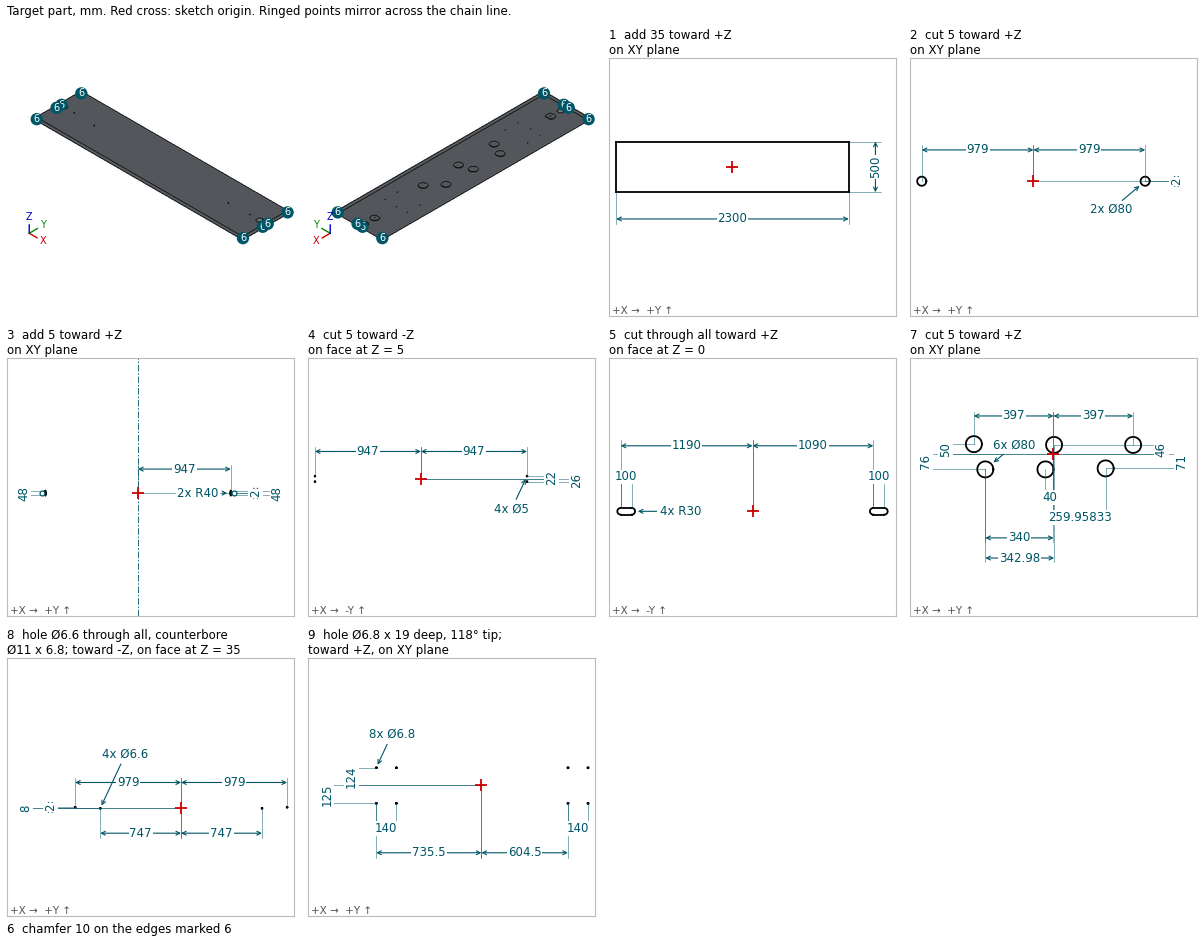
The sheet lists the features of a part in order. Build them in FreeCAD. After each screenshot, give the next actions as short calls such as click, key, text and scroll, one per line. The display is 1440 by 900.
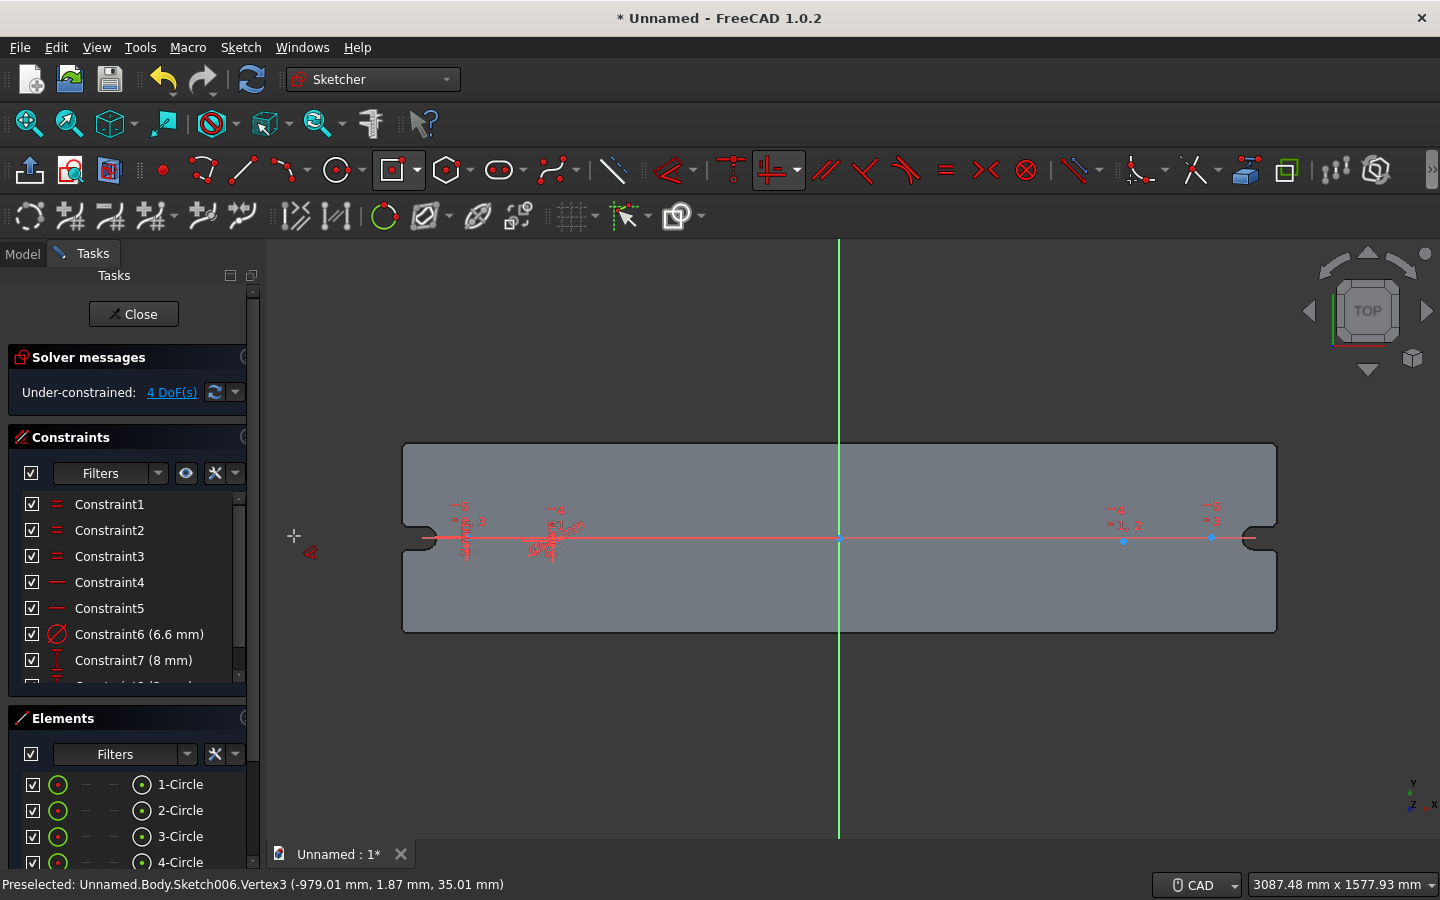
click(555, 541)
click(697, 575)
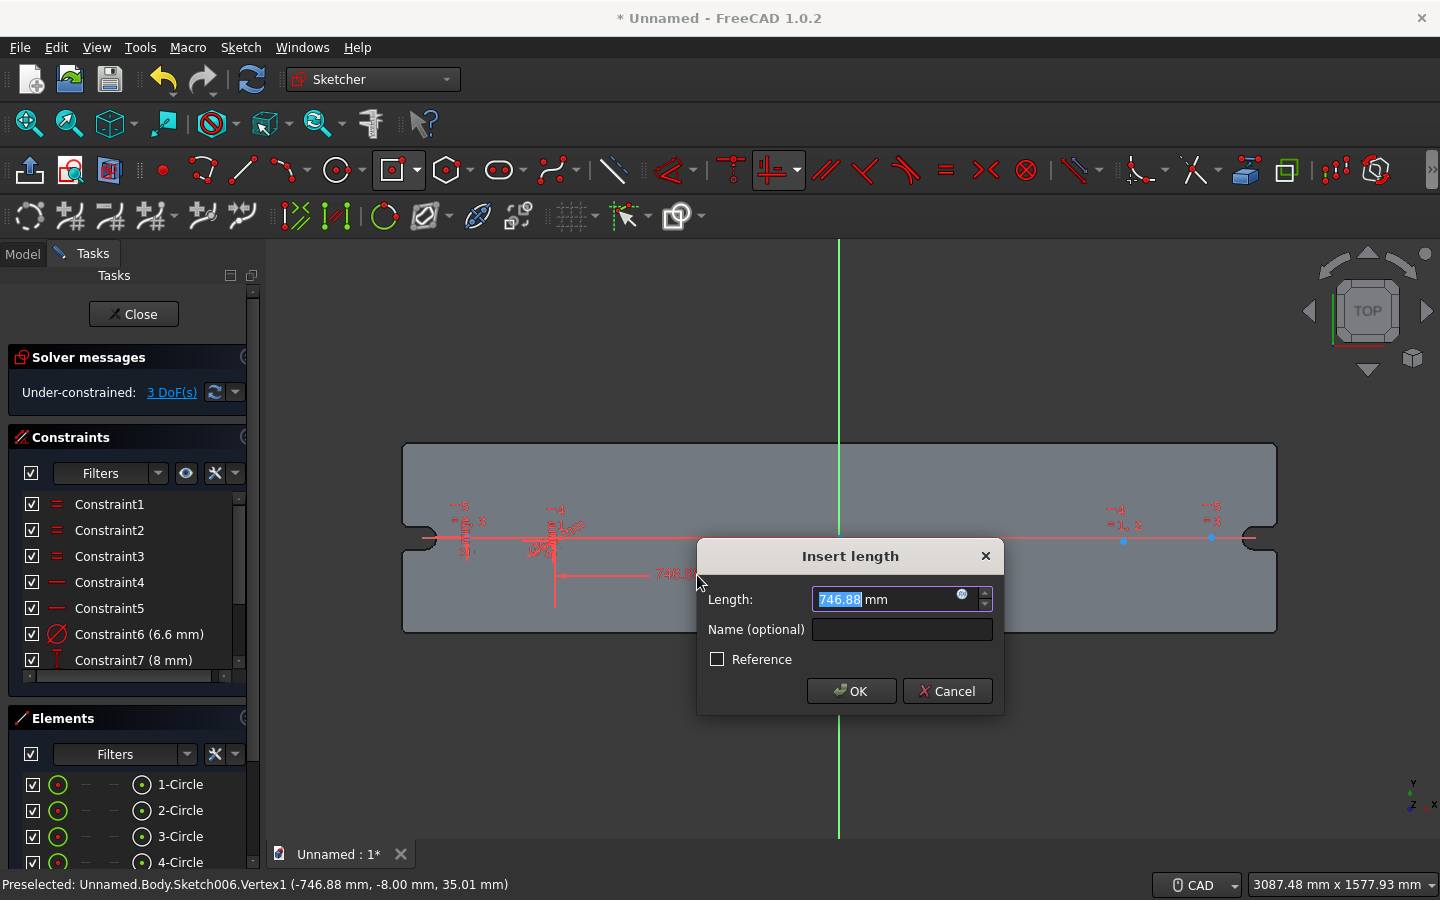
text(747)
key(Return)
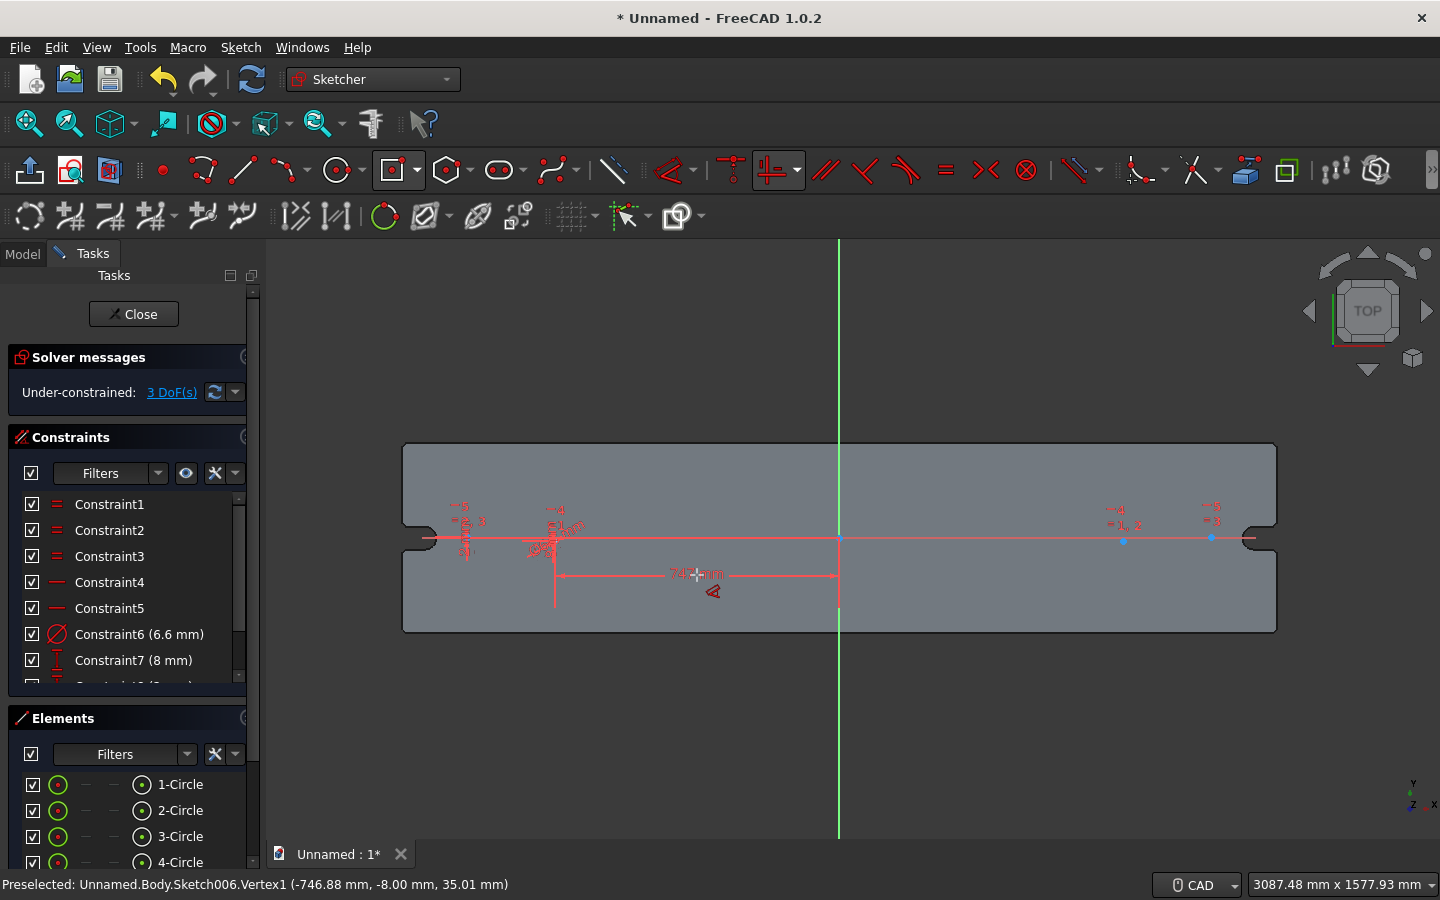
click(1123, 541)
click(981, 575)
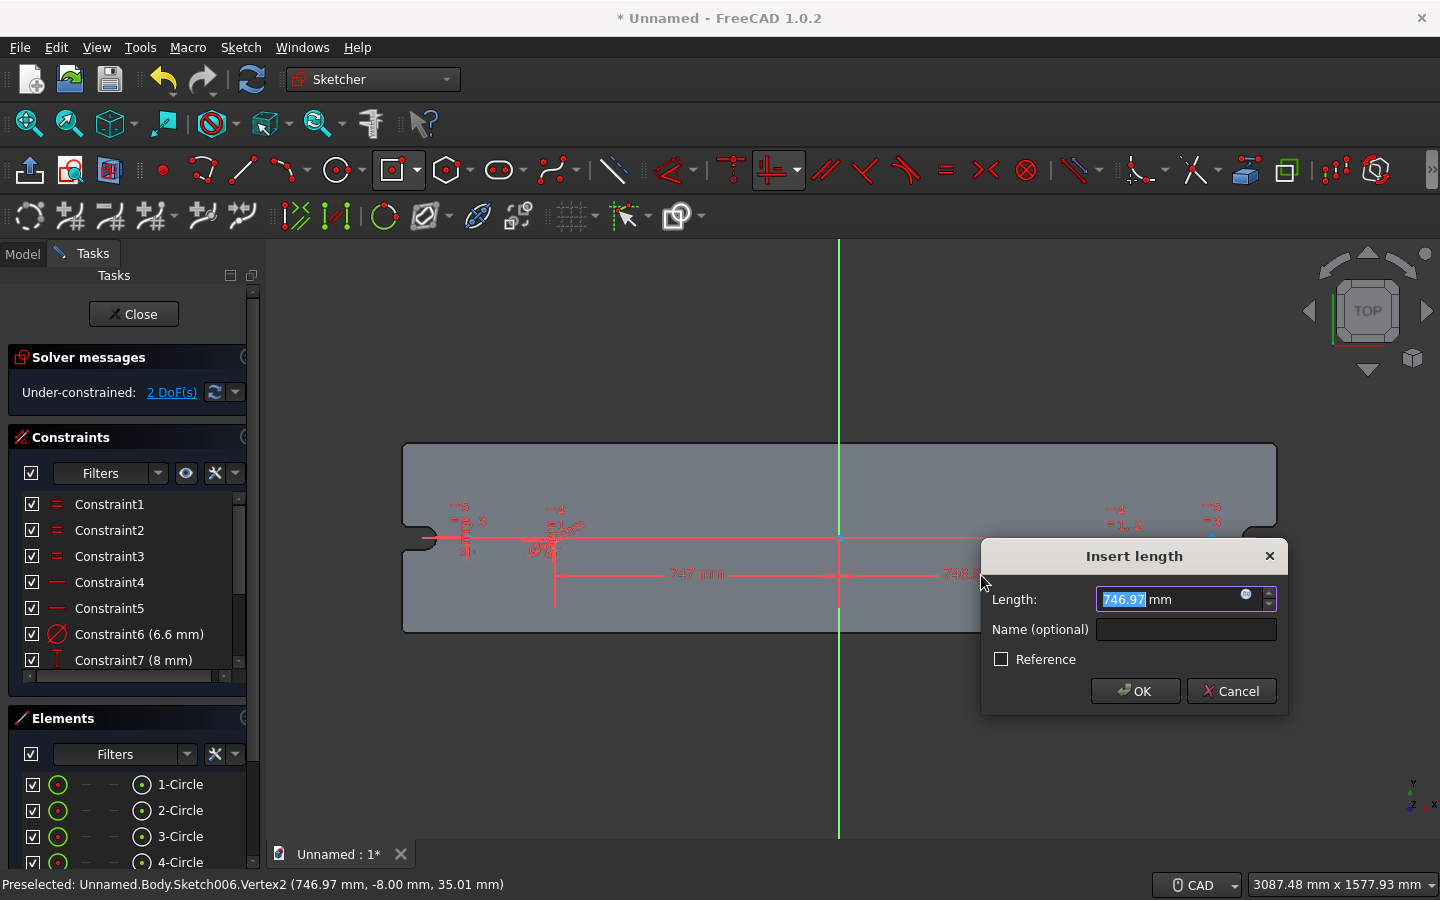
text(747)
key(Return)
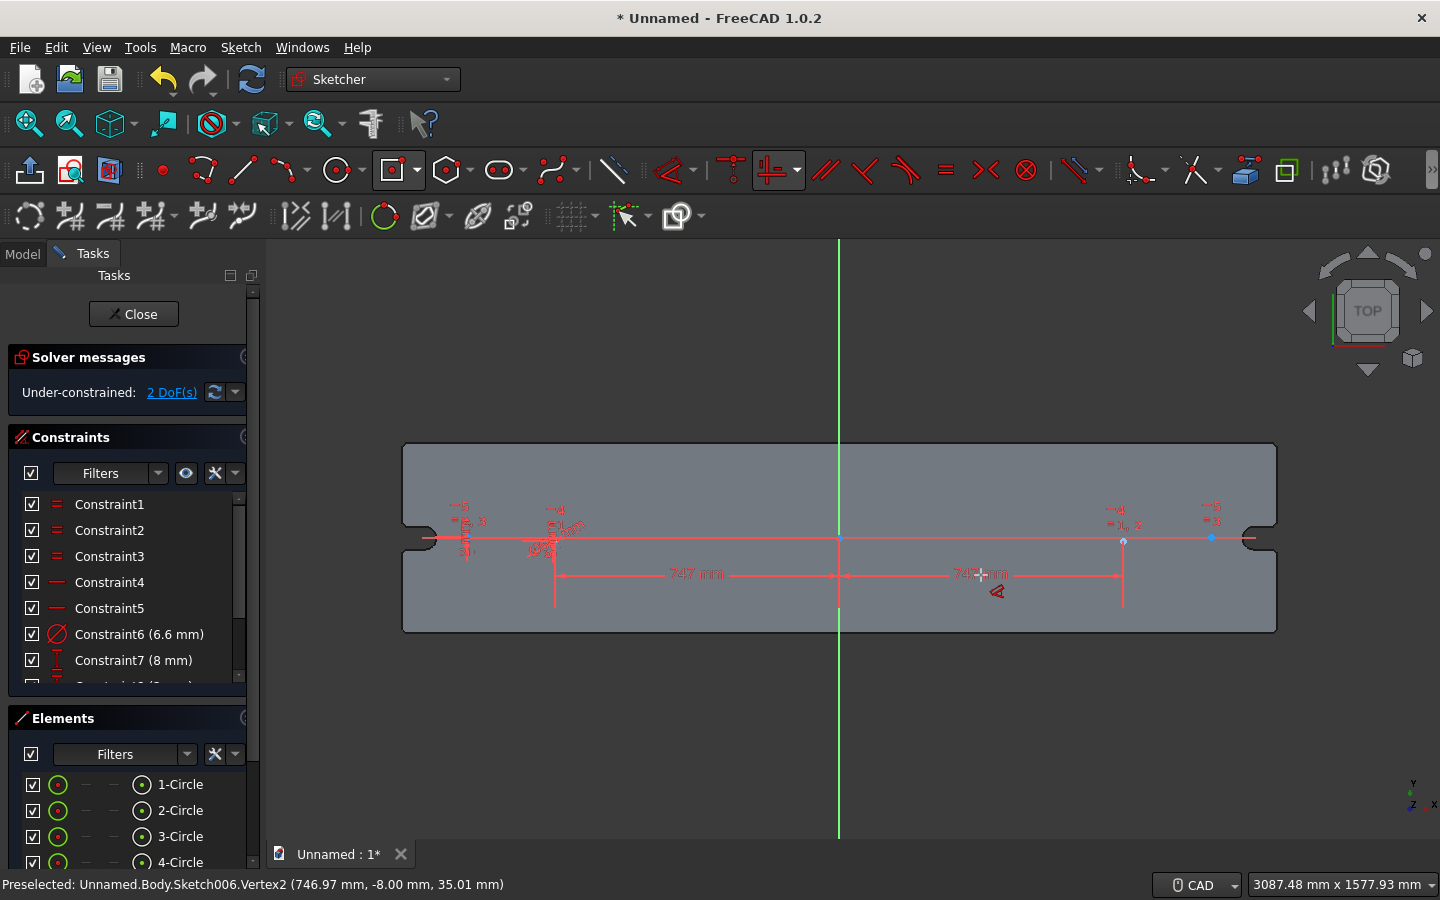
click(467, 537)
click(653, 503)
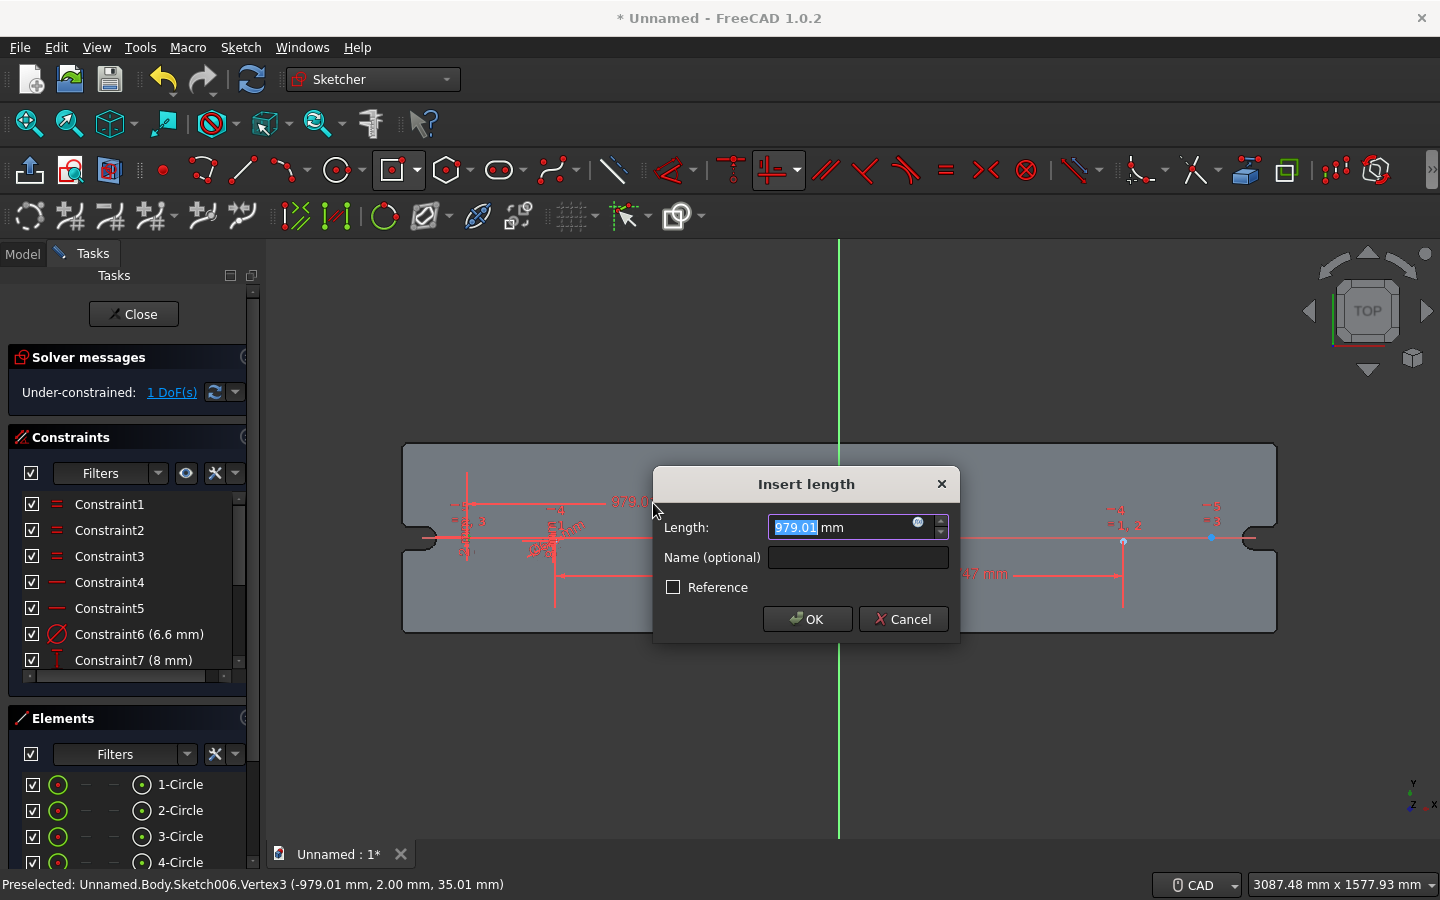
text(979)
key(Return)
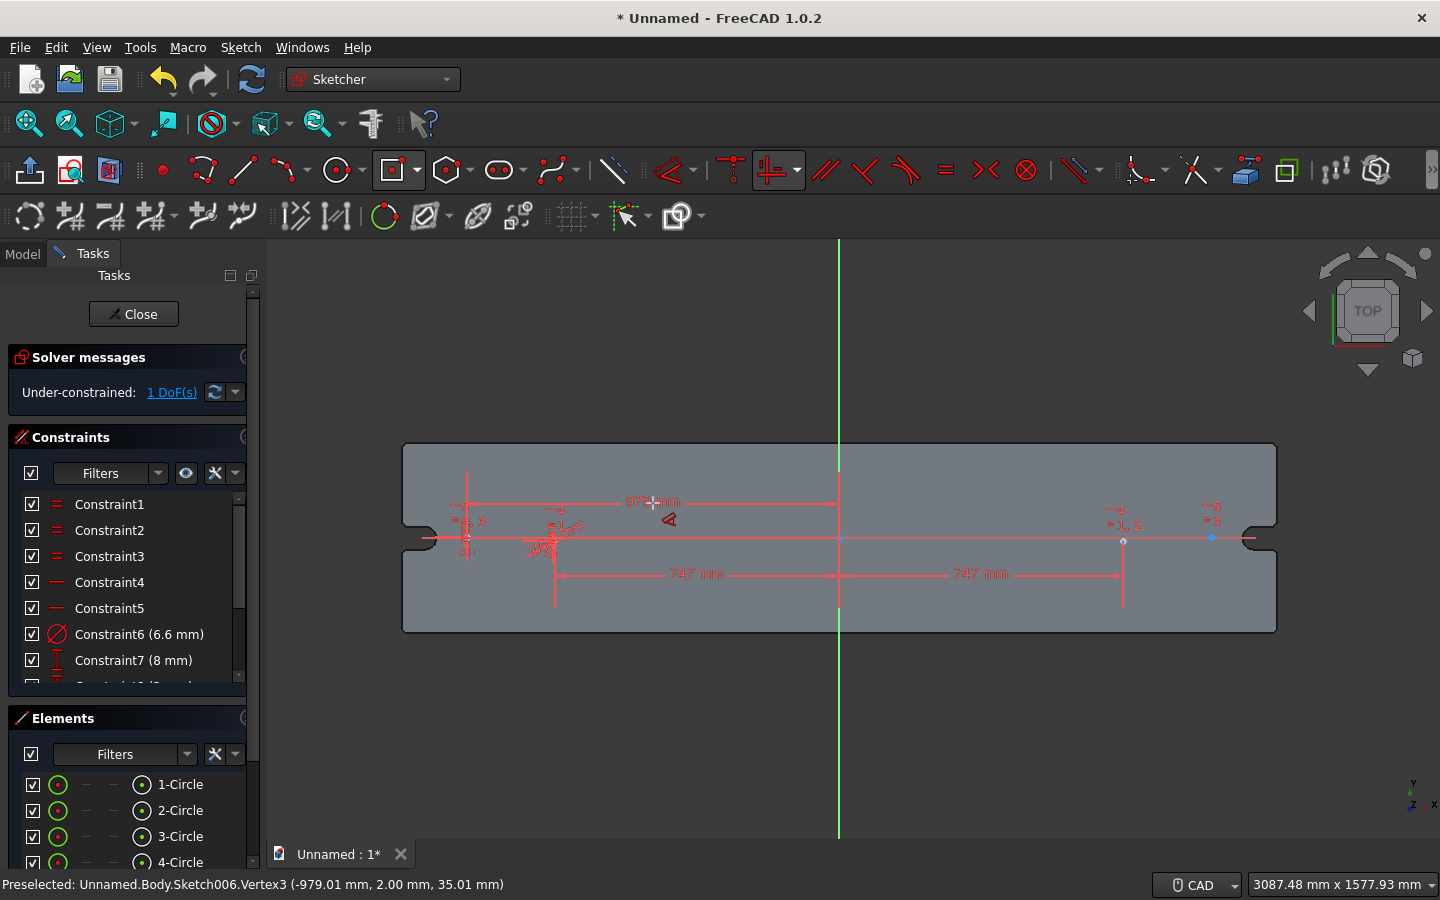
click(1212, 537)
click(1026, 503)